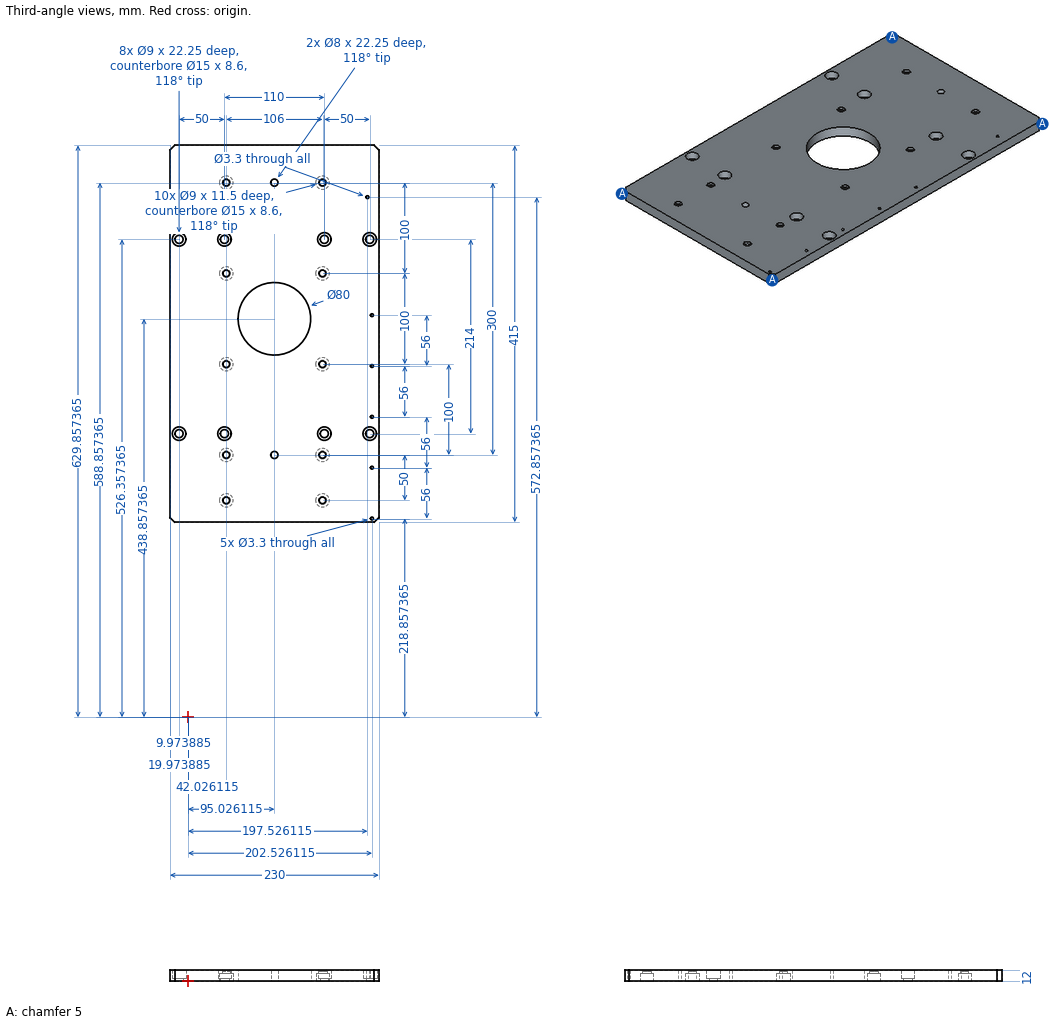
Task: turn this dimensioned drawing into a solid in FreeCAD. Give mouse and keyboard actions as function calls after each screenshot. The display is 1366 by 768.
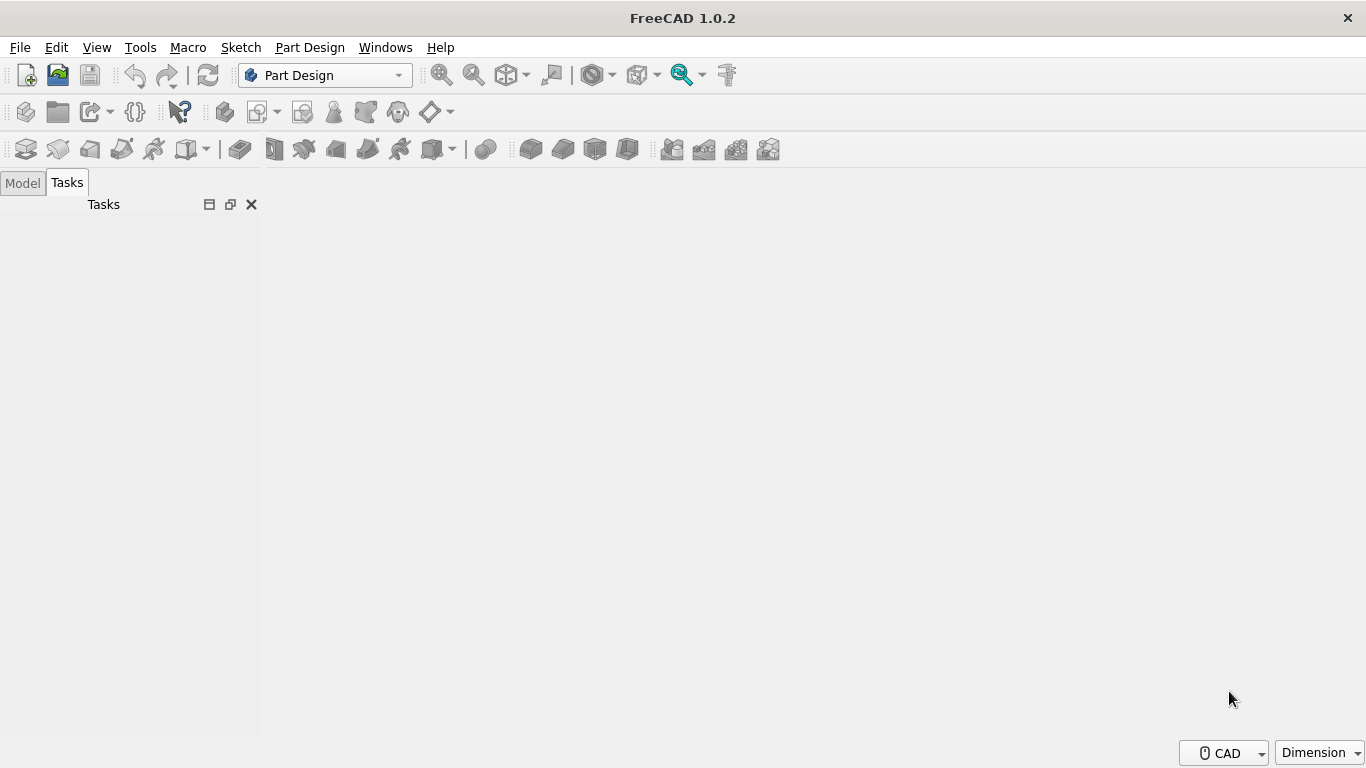
click(702, 76)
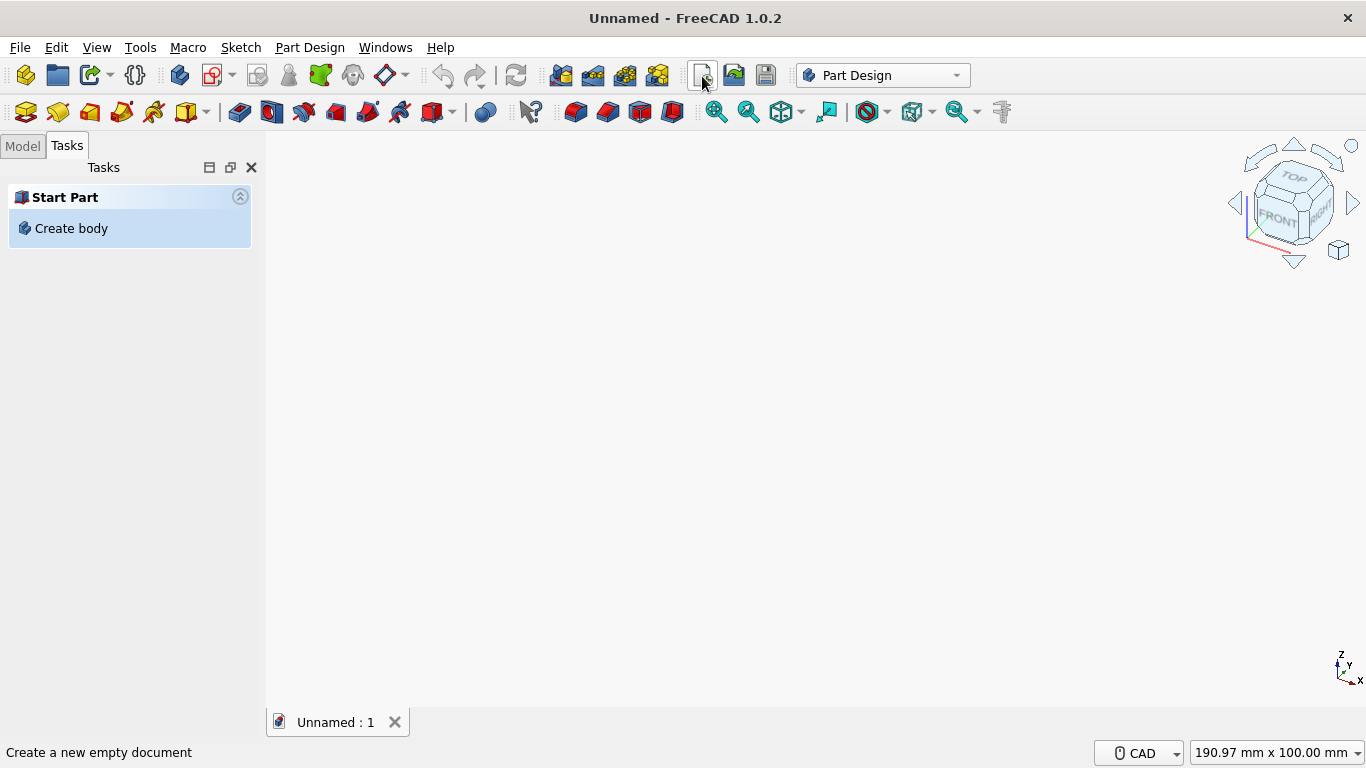
click(212, 76)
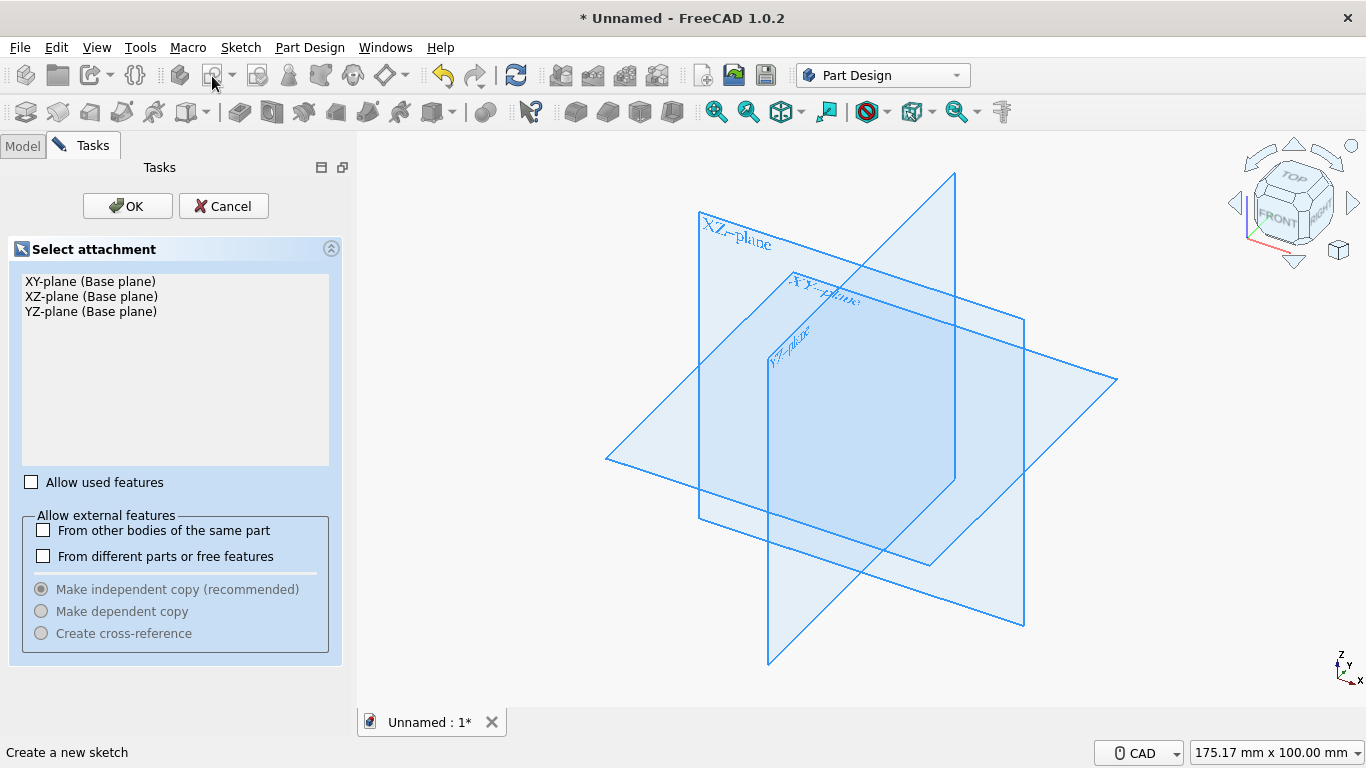
click(82, 282)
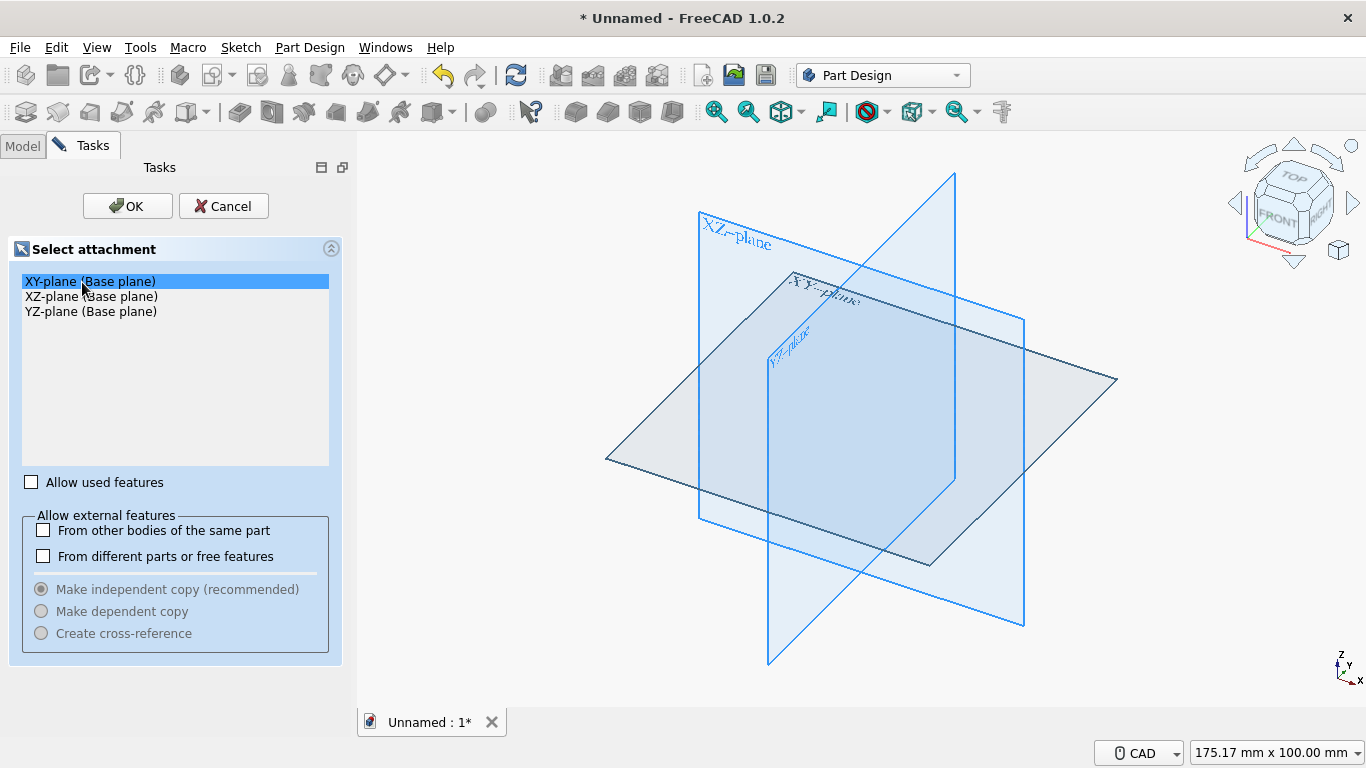
click(128, 206)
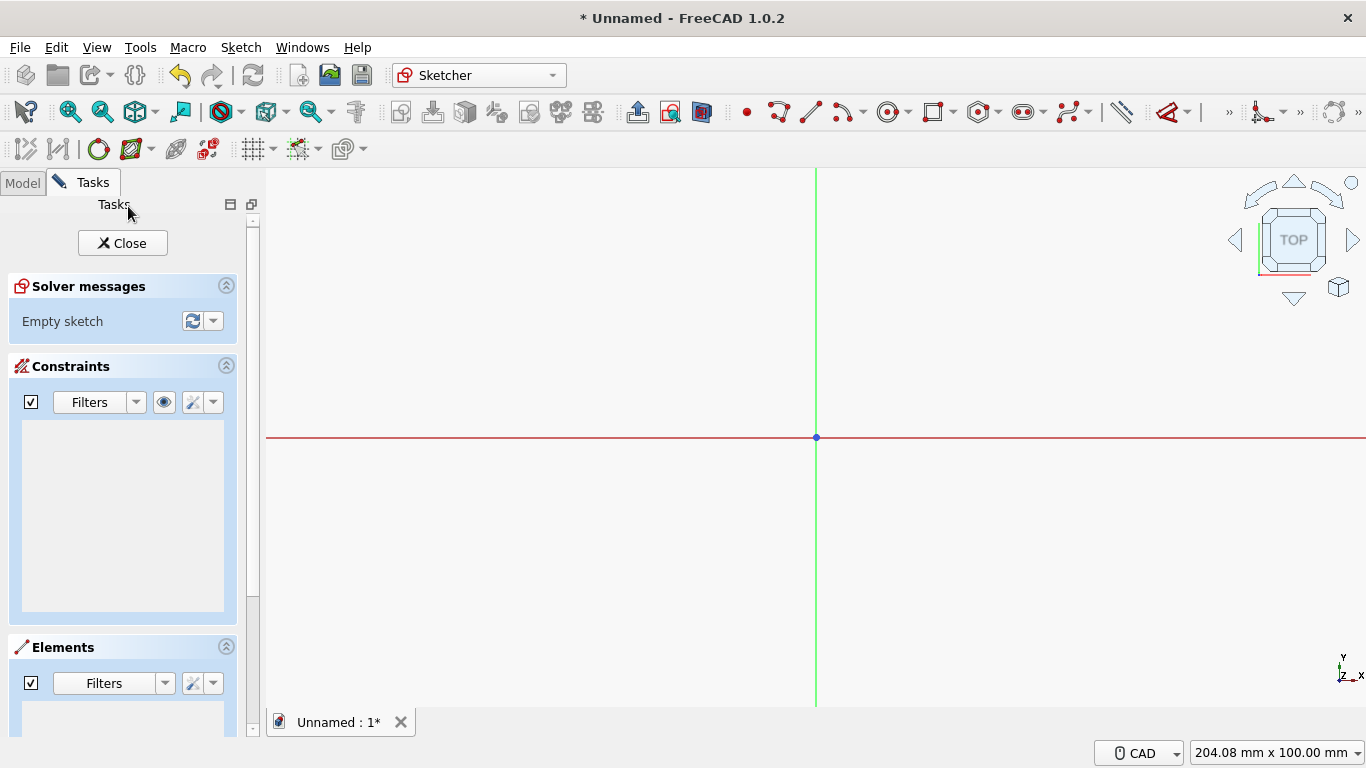
scroll(675, 649, down, 11)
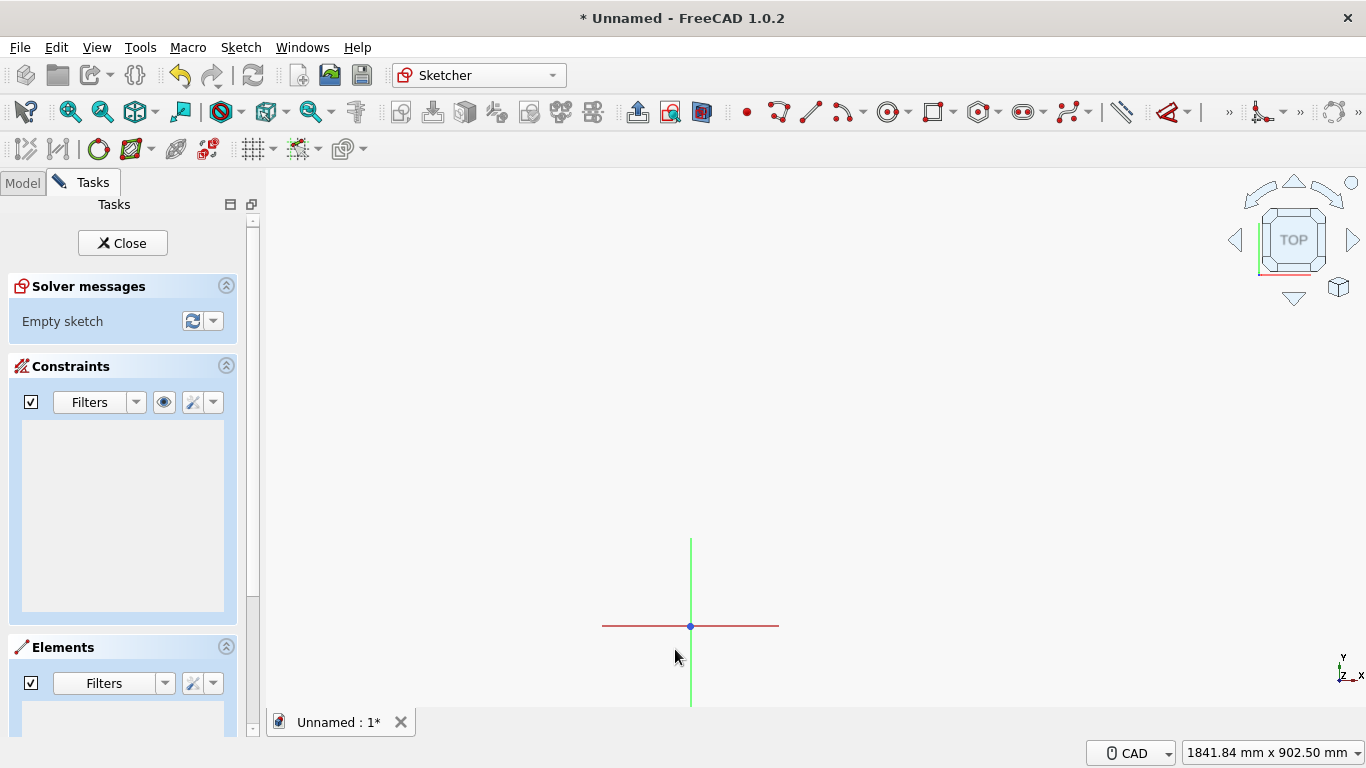
click(934, 112)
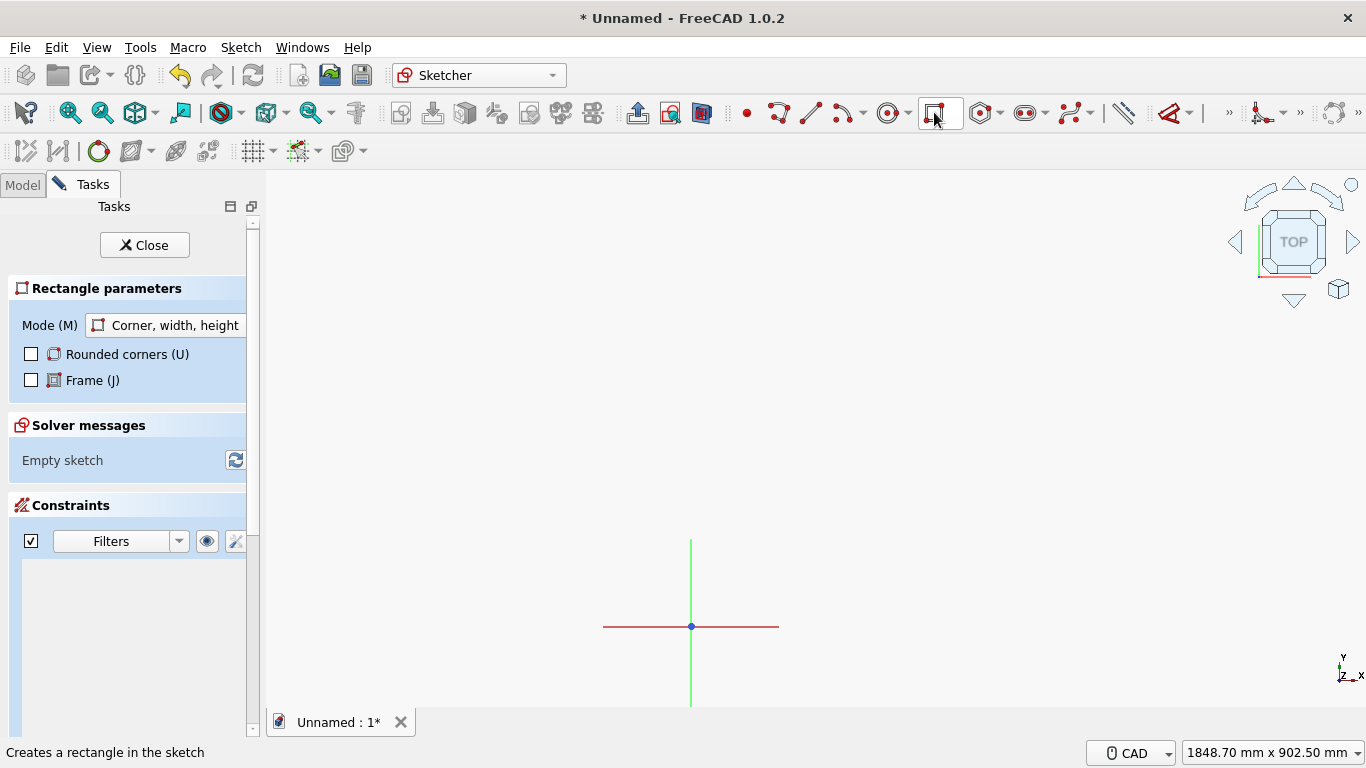
scroll(680, 252, up, 2)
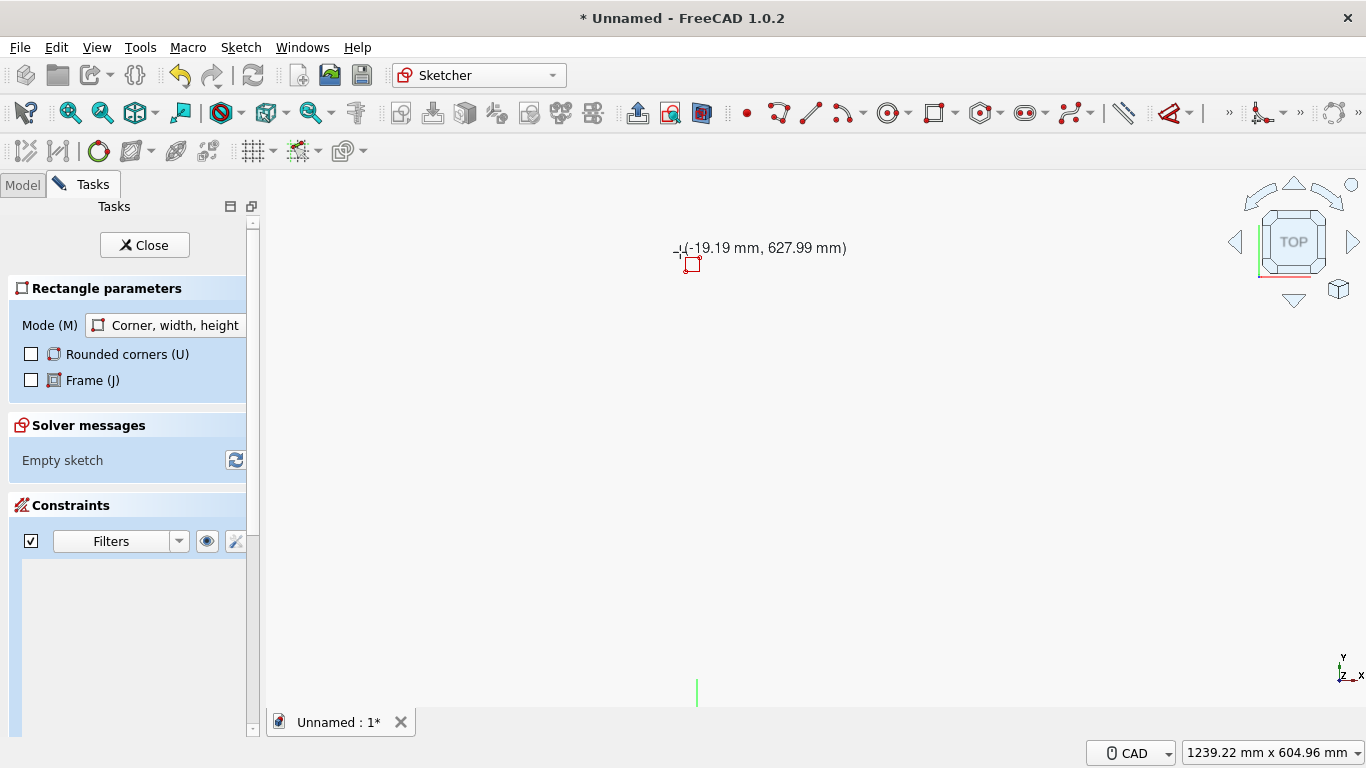
click(679, 252)
move(883, 620)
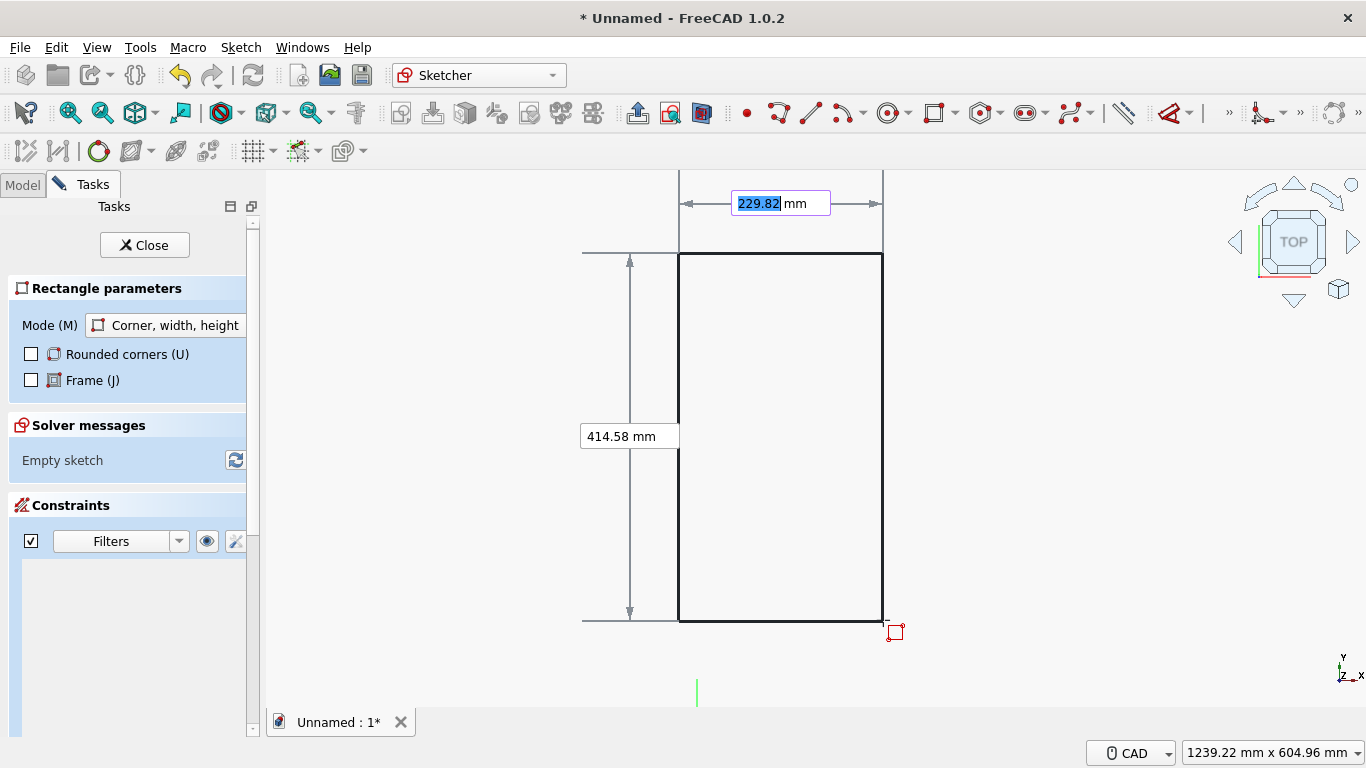
text(230)
key(Tab)
text(415)
key(Return)
key(Escape)